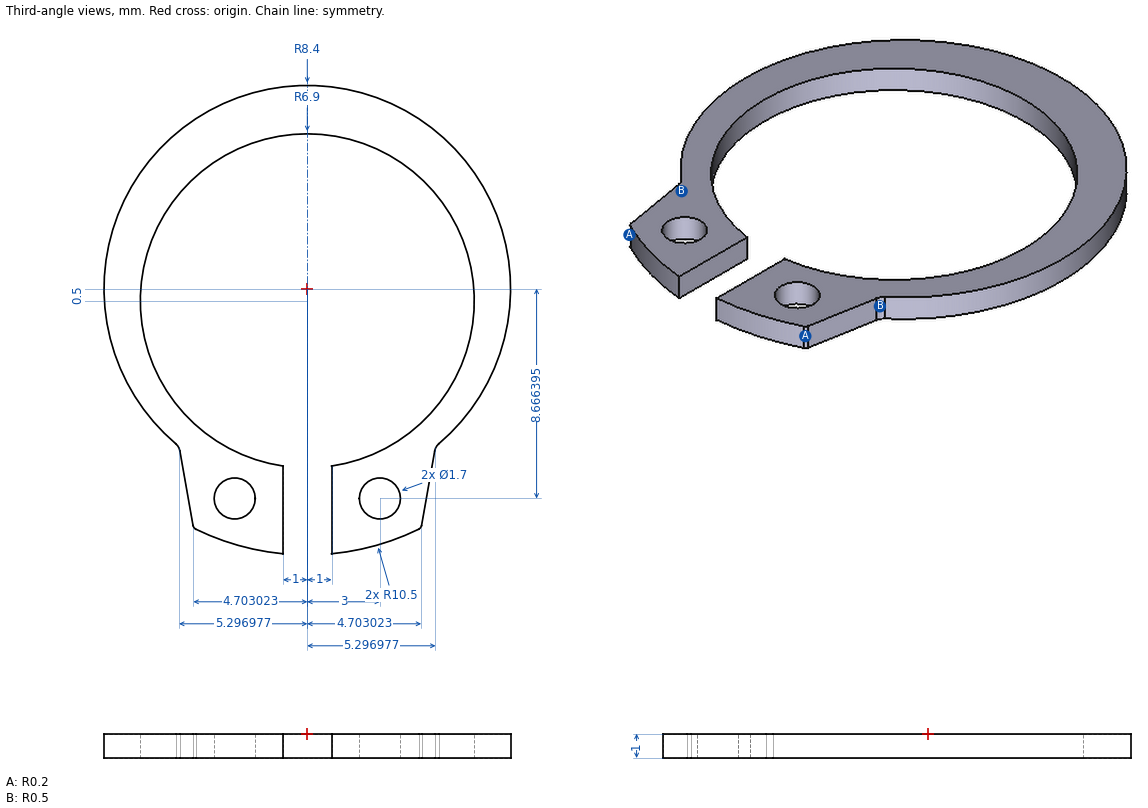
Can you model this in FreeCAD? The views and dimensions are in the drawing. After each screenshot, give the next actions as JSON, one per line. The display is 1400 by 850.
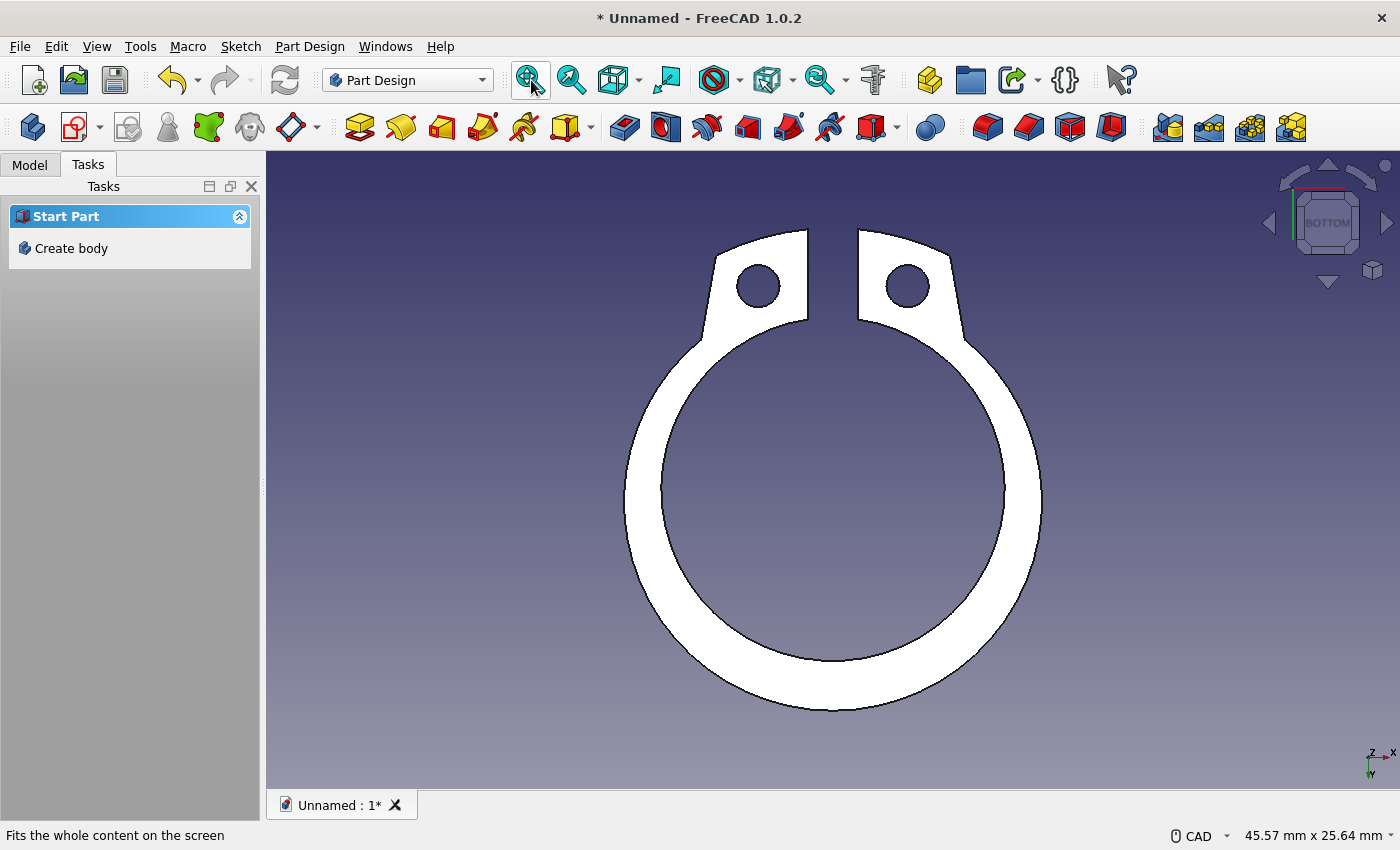
{"action": "key", "text": "4"}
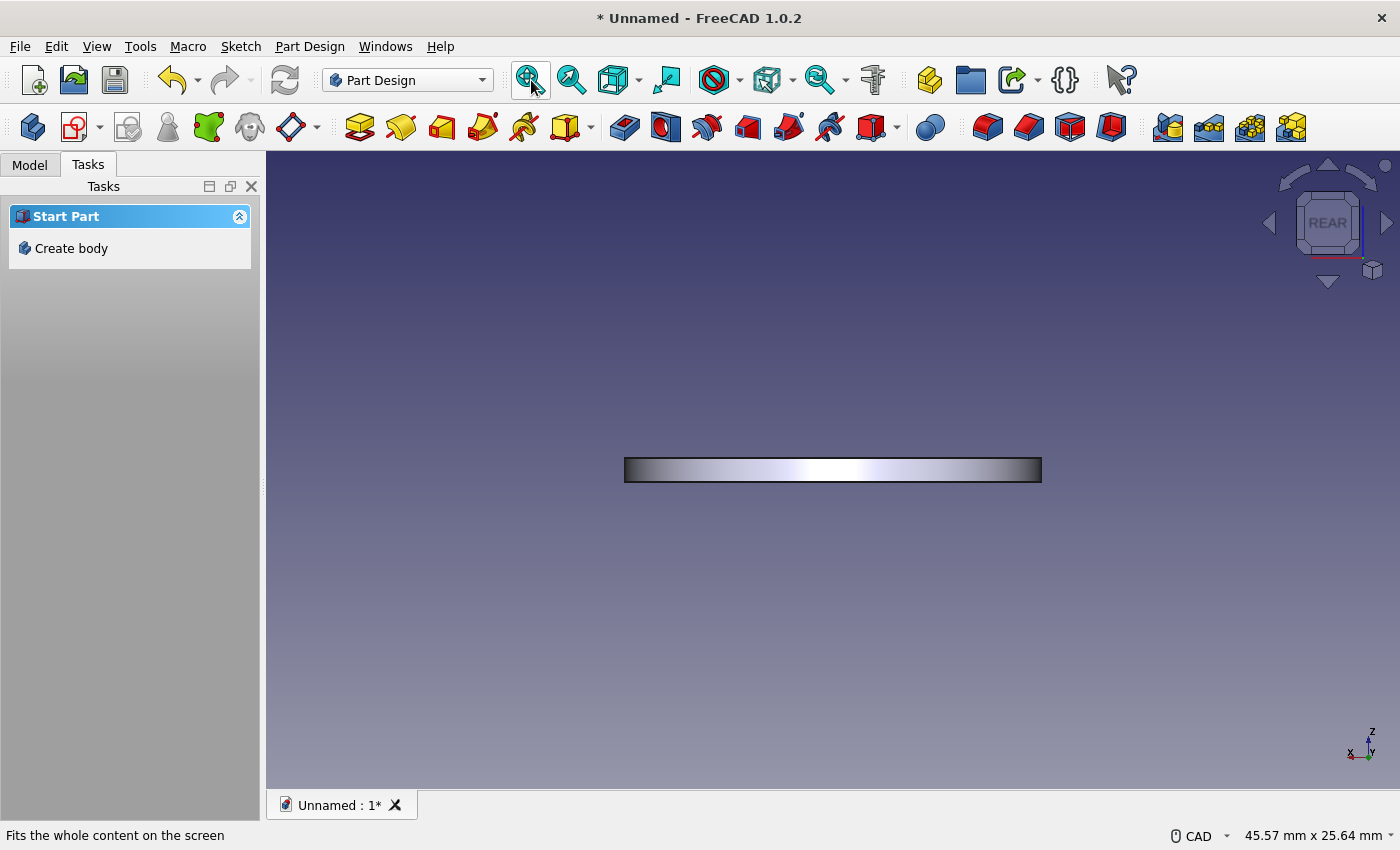
{"action": "left_click", "coordinate": [531, 80]}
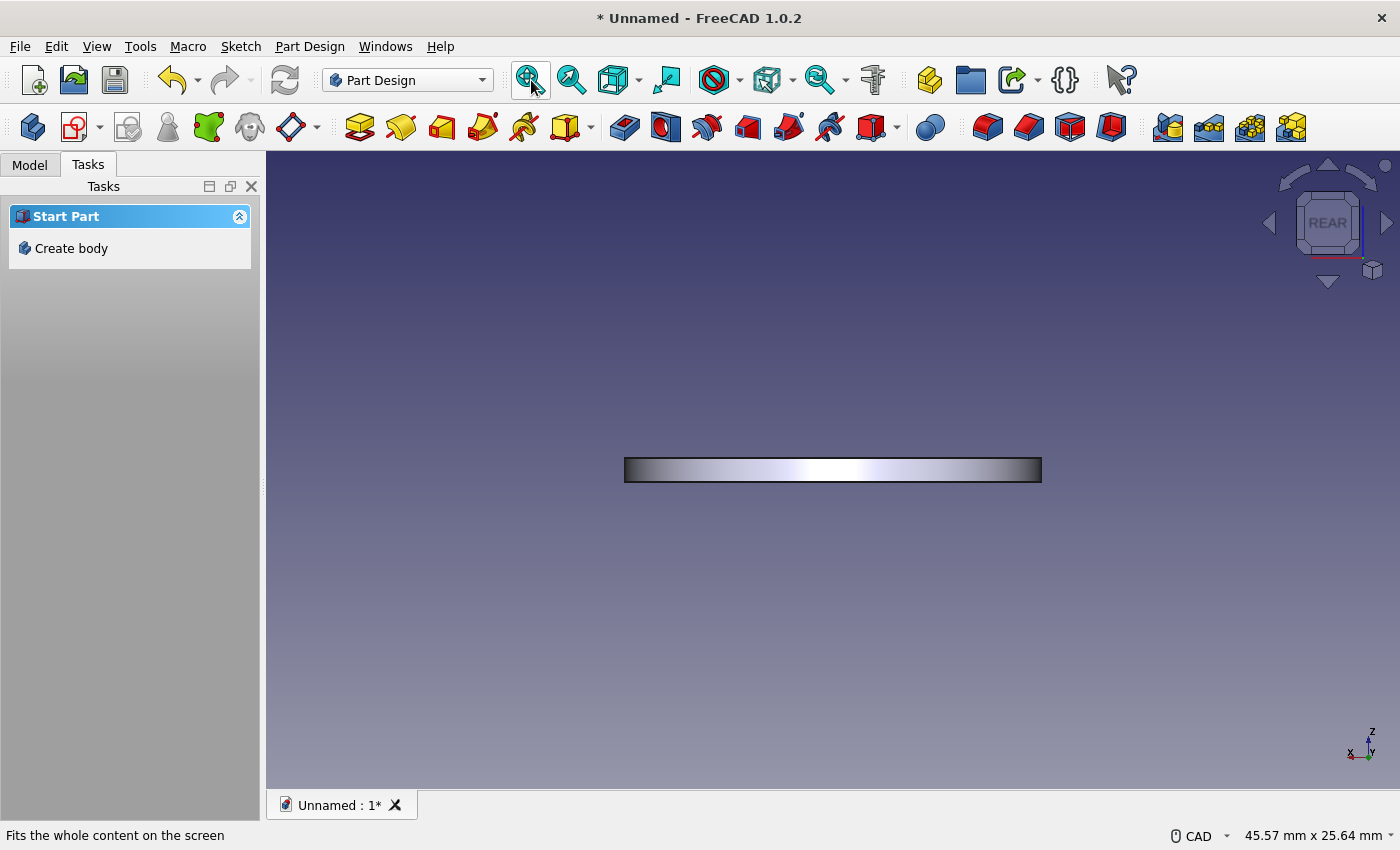
{"action": "key", "text": "6"}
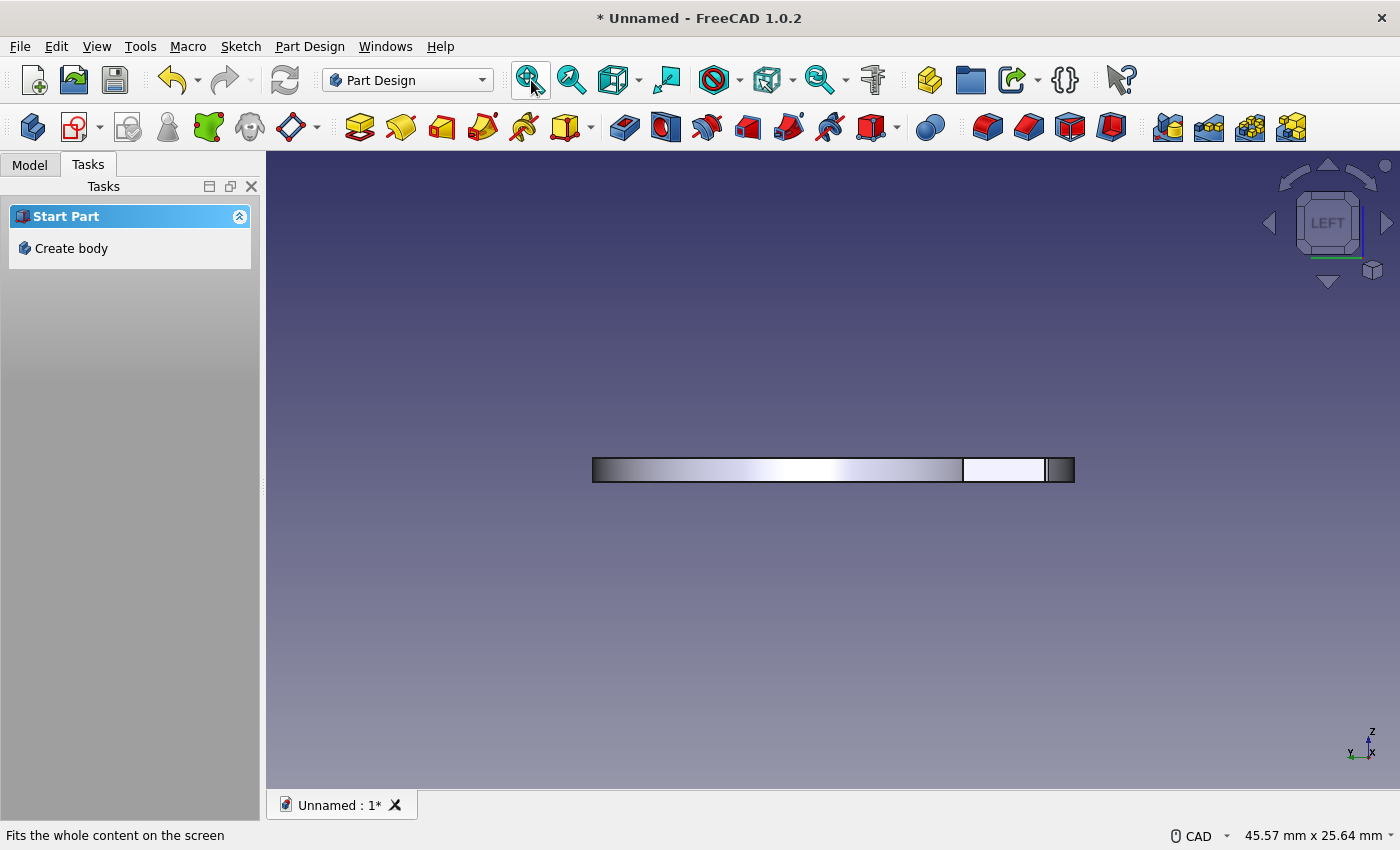
{"action": "left_click", "coordinate": [531, 80]}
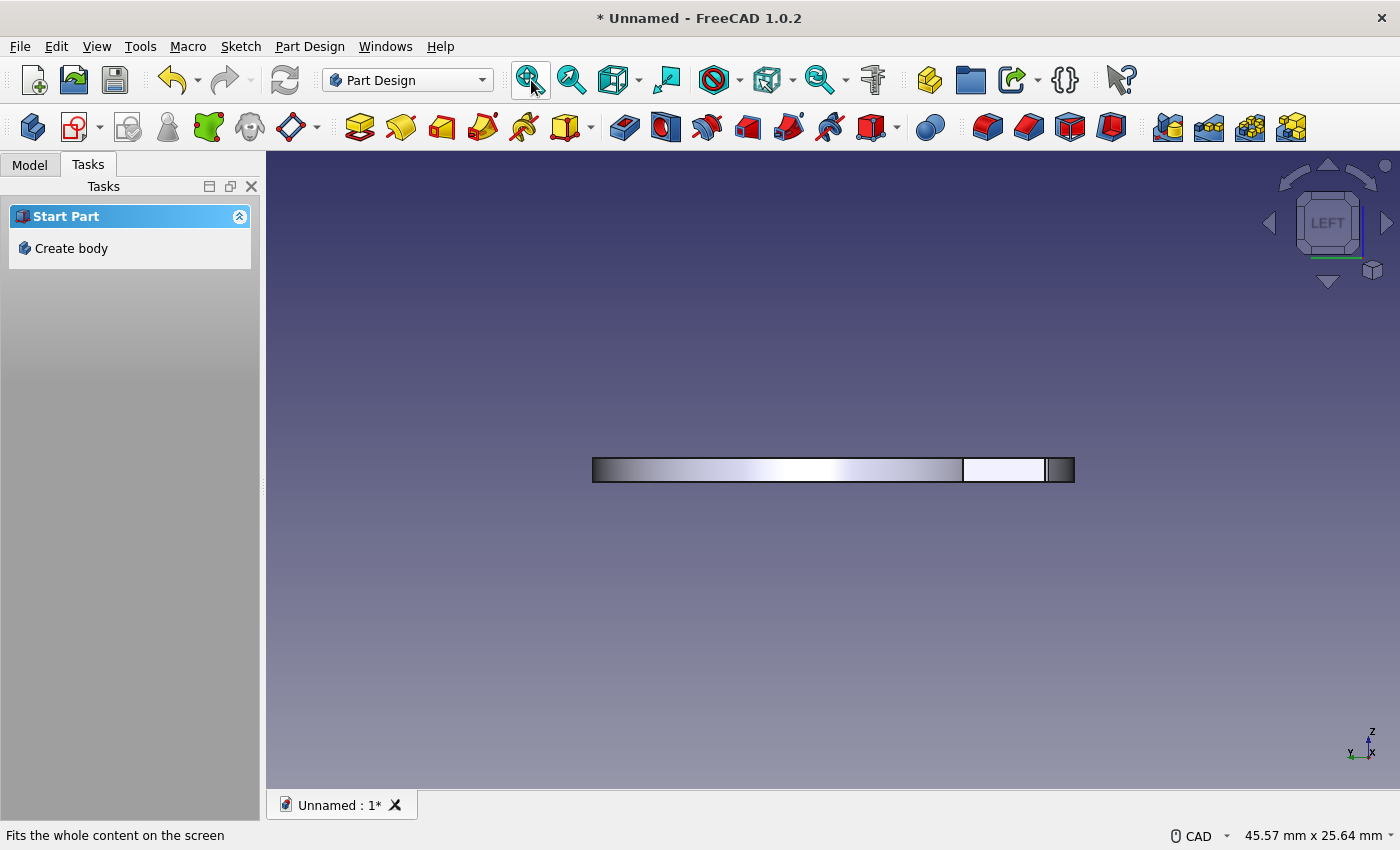
{"action": "key", "text": "v 3"}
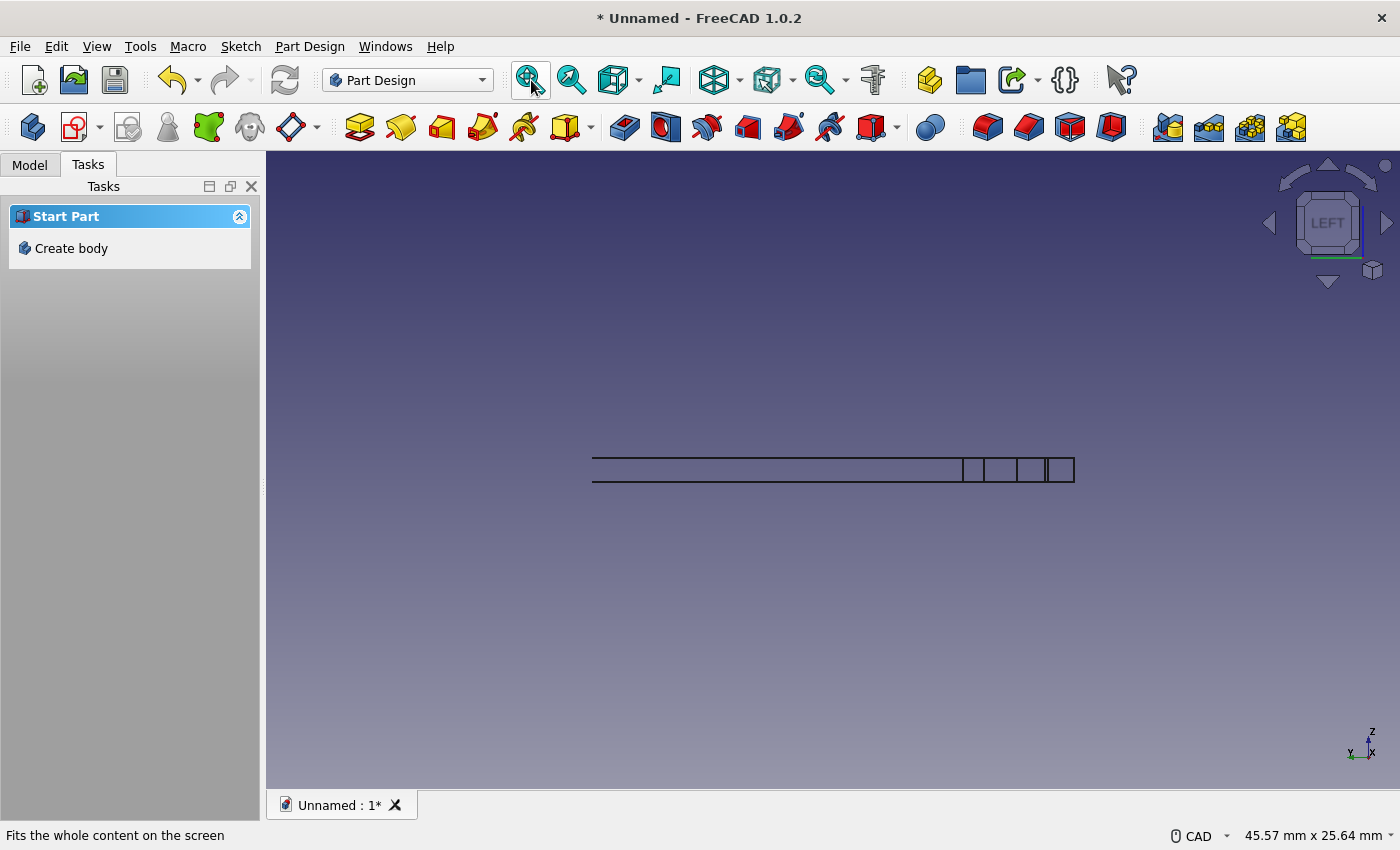
{"action": "key", "text": "0"}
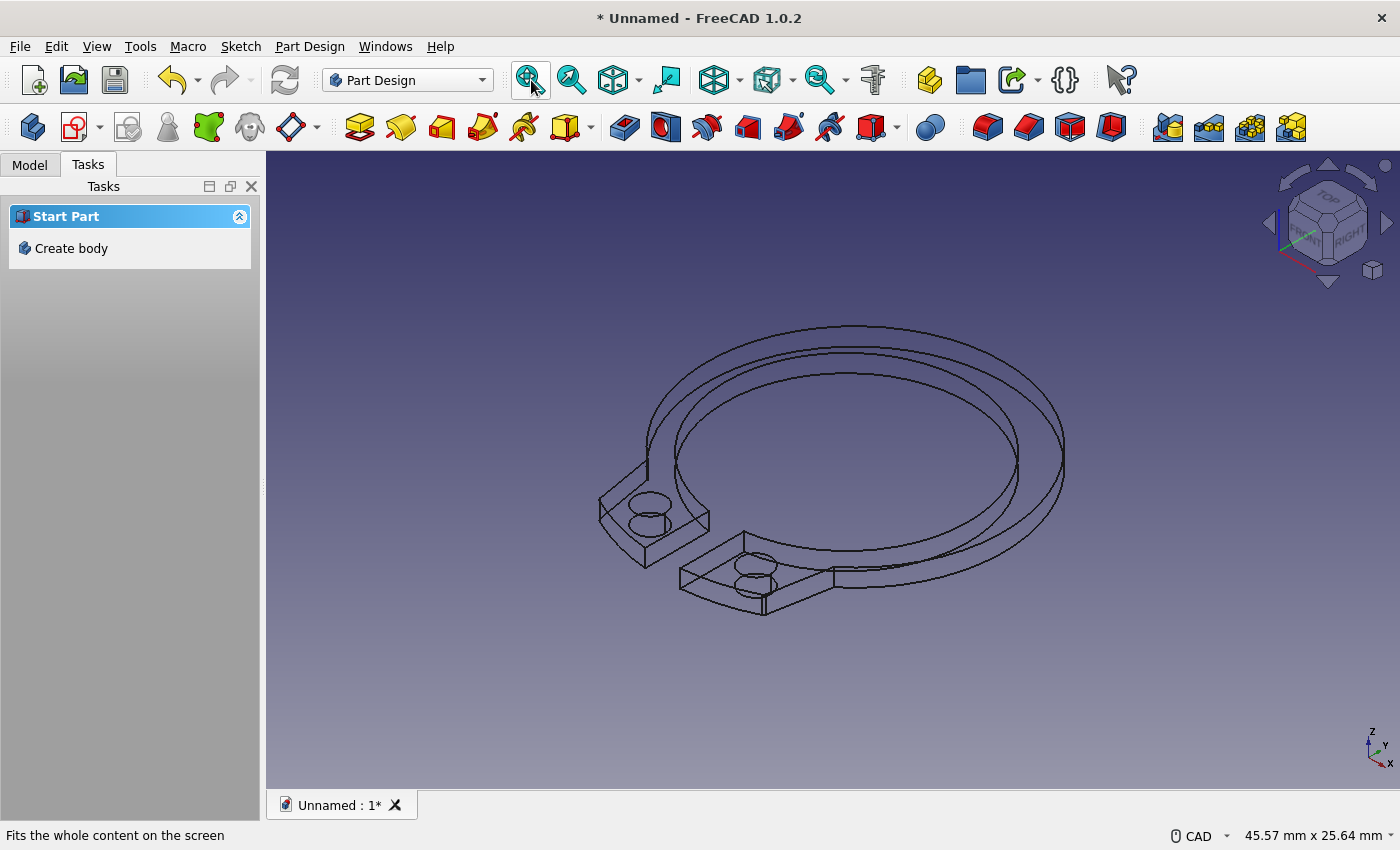
{"action": "left_click", "coordinate": [648, 468]}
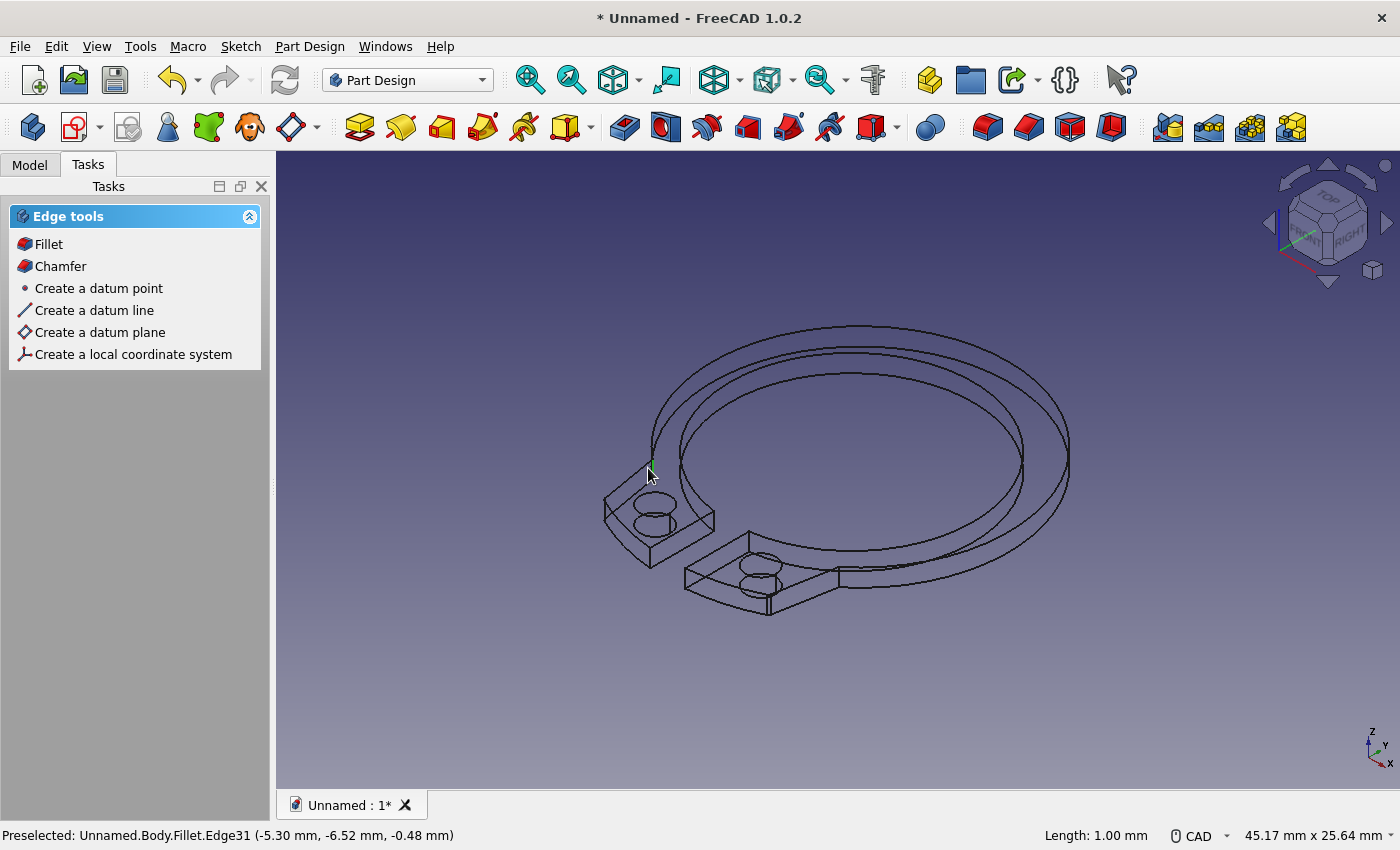
{"action": "left_click", "coordinate": [839, 576], "text": "ctrl"}